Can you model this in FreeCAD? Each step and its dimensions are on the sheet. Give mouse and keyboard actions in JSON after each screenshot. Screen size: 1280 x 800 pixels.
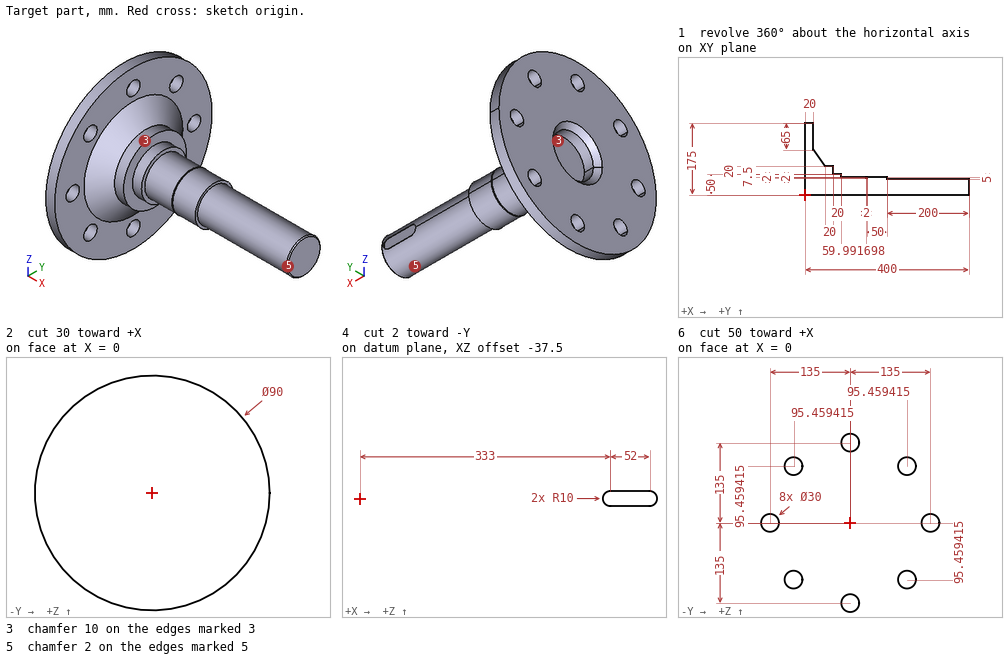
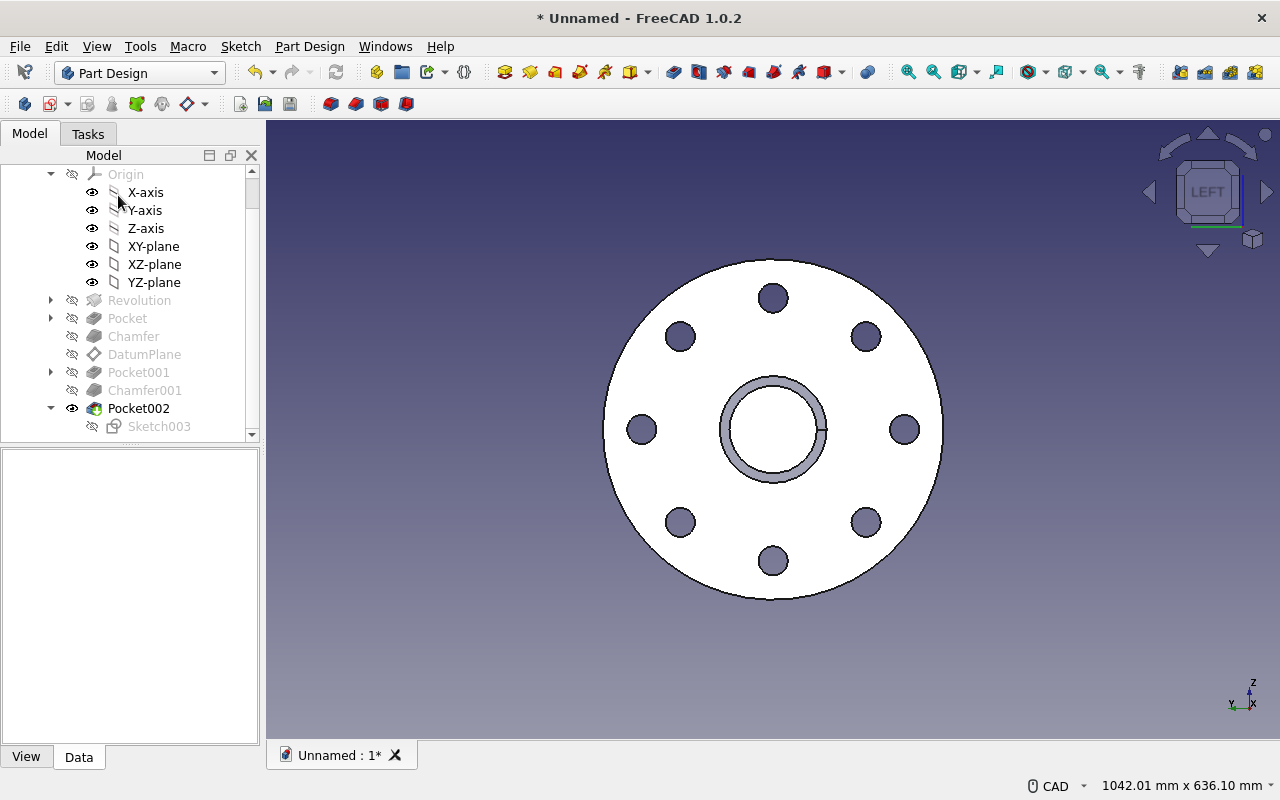
{"action": "key", "text": "0"}